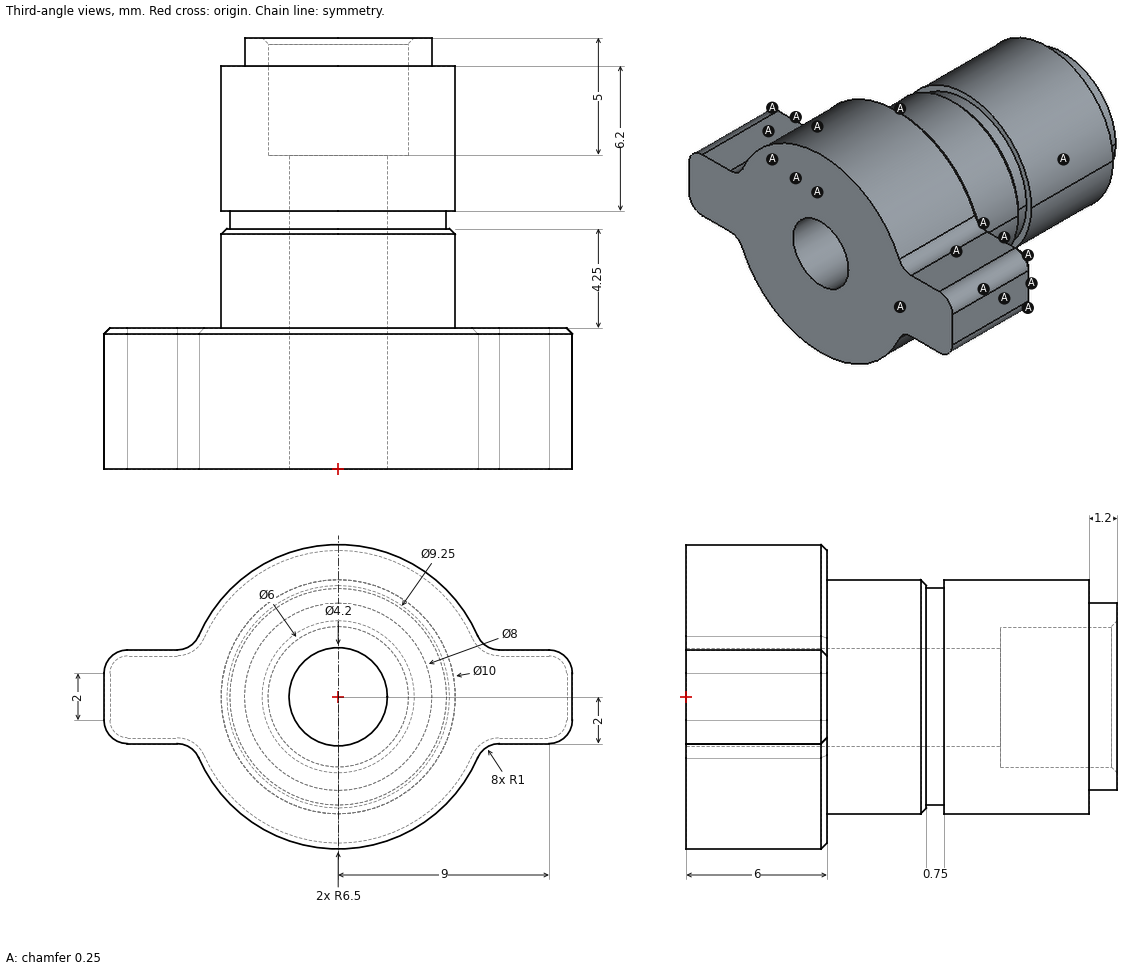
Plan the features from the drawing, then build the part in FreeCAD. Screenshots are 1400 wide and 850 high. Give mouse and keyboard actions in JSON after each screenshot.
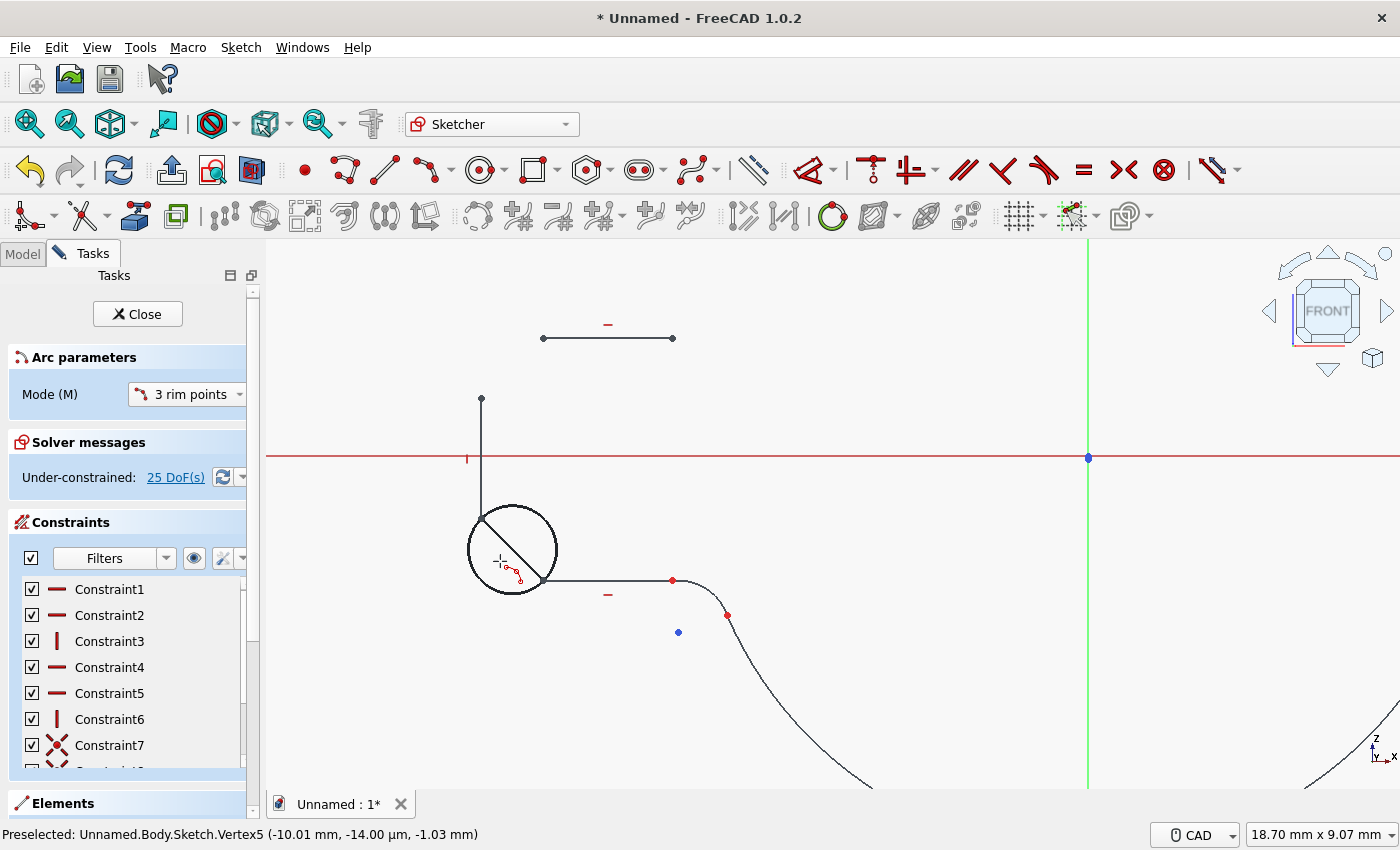
{"action": "left_click", "coordinate": [500, 560]}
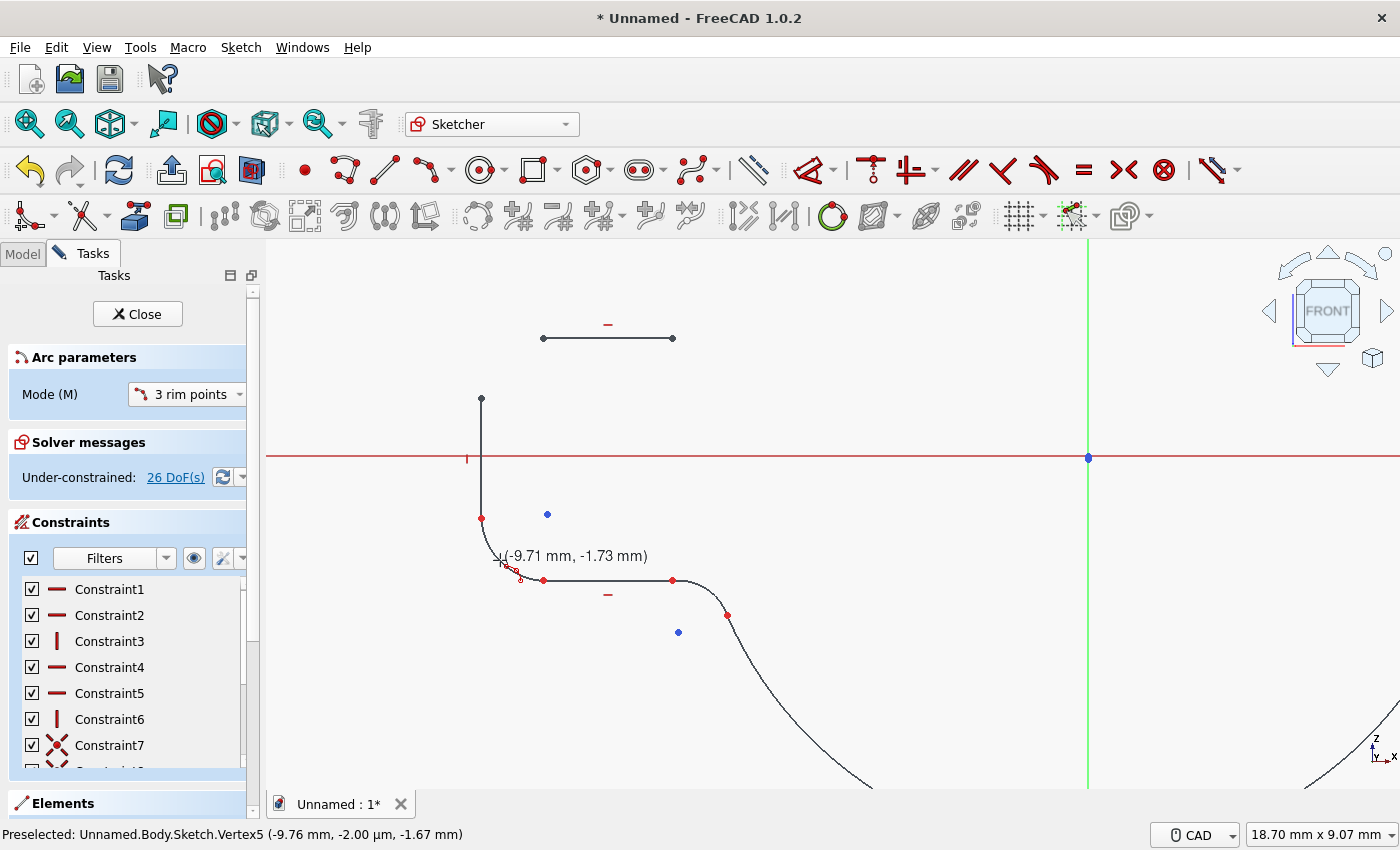
{"action": "left_click", "coordinate": [481, 398]}
{"action": "left_click", "coordinate": [544, 338]}
{"action": "left_click", "coordinate": [500, 353]}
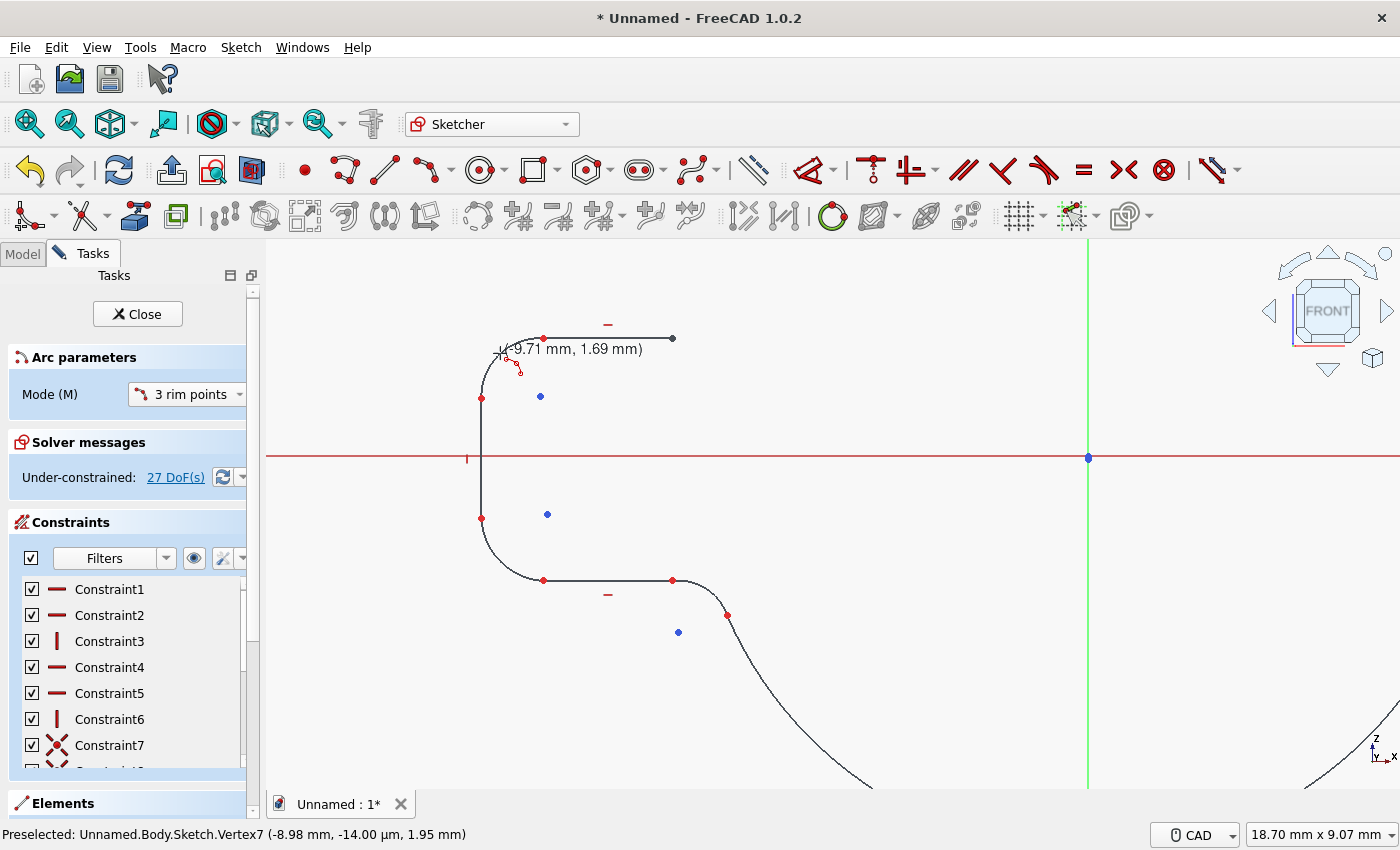
{"action": "left_click", "coordinate": [673, 338]}
{"action": "left_click", "coordinate": [727, 299]}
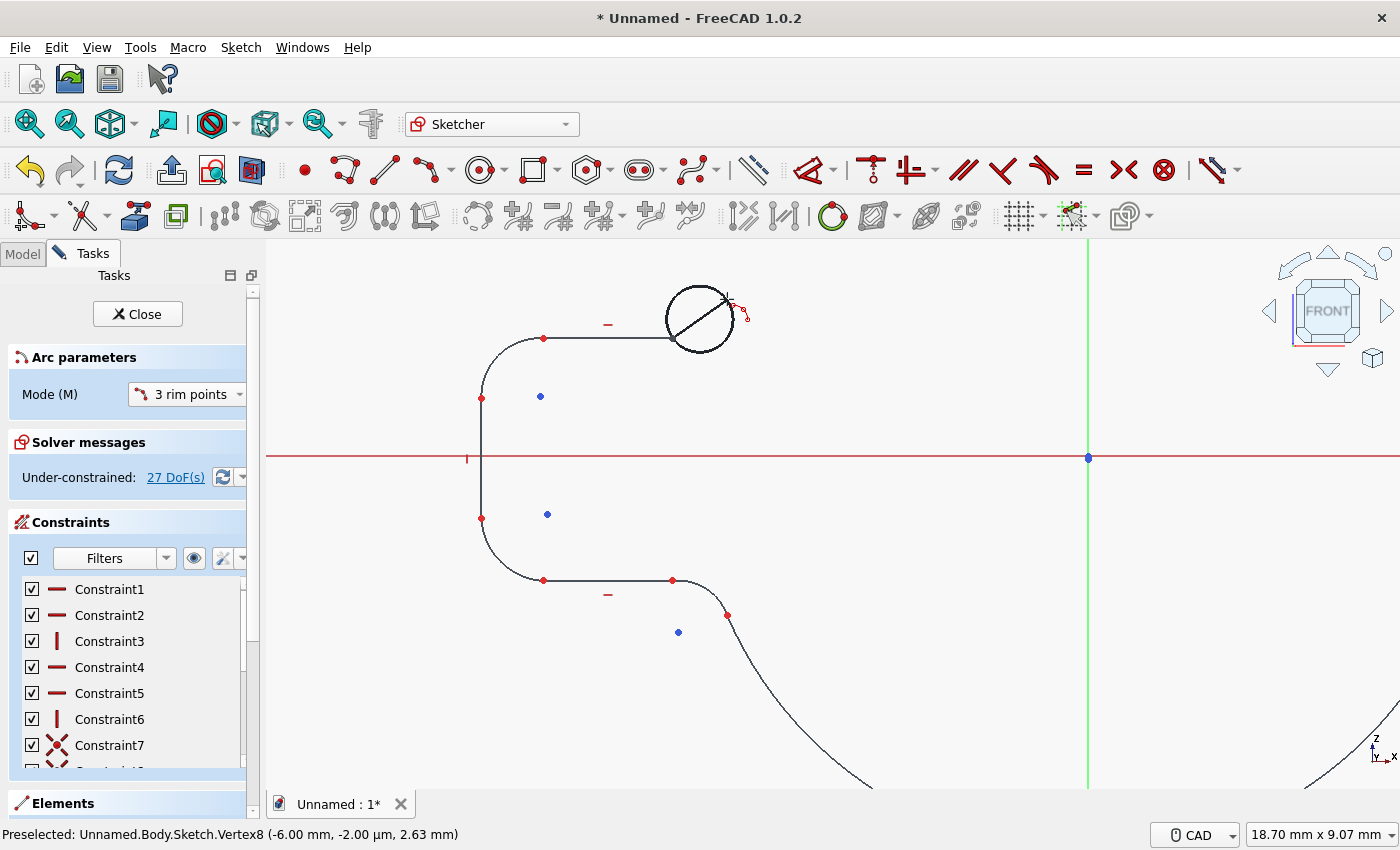
{"action": "scroll", "coordinate": [705, 325], "scroll_direction": "up", "scroll_amount": 3}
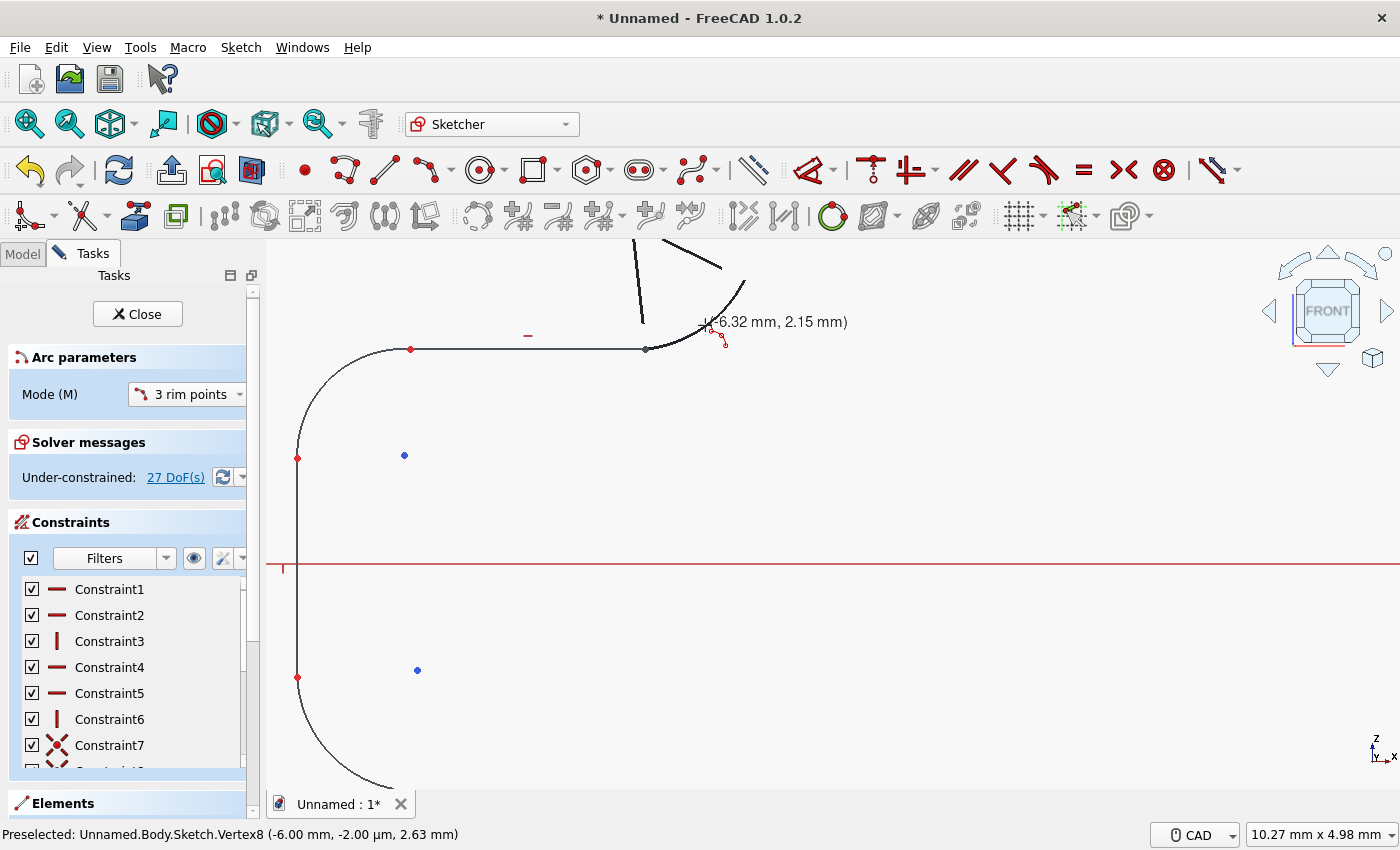
{"action": "left_click", "coordinate": [704, 325]}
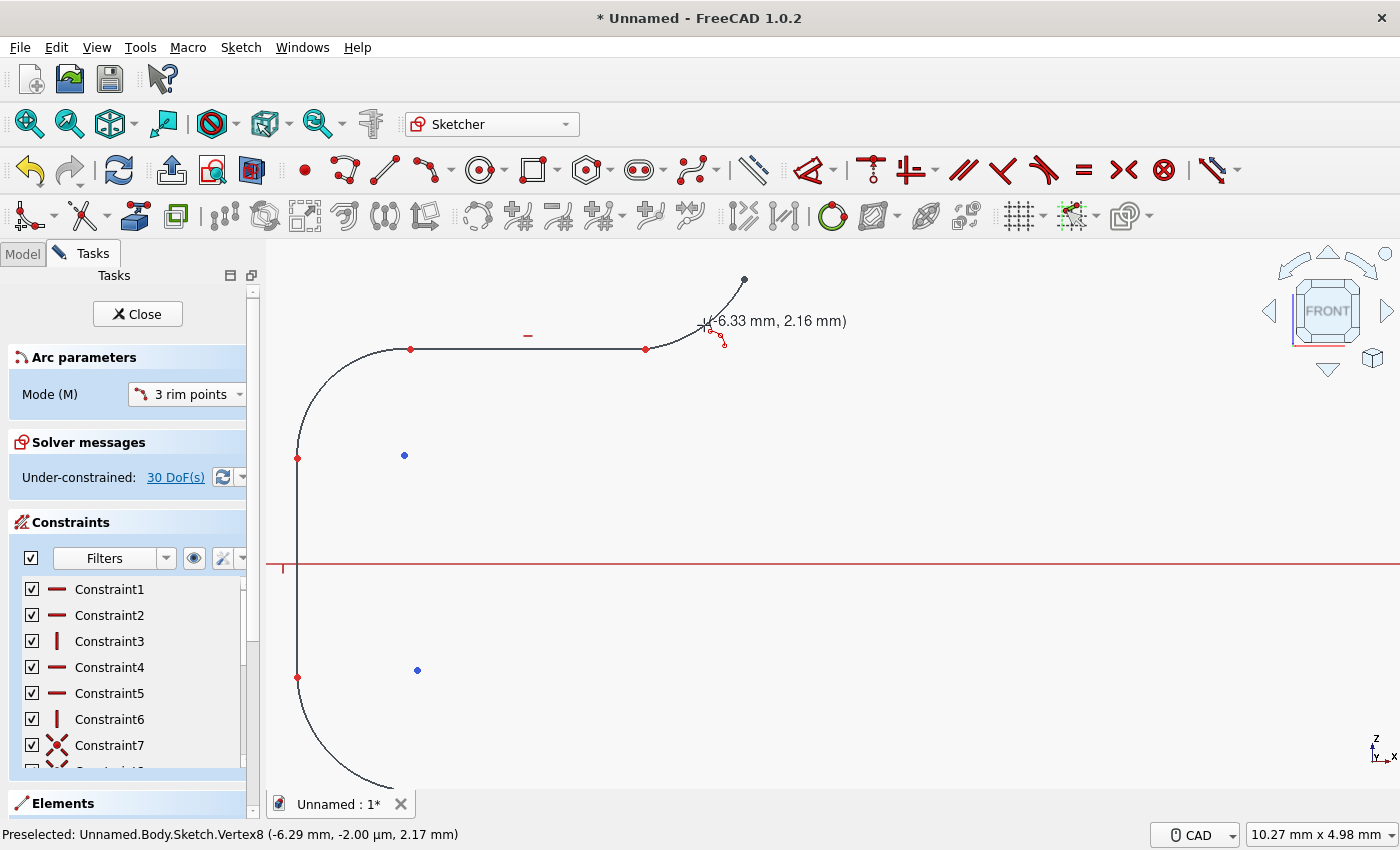
{"action": "scroll", "coordinate": [555, 498], "scroll_direction": "down", "scroll_amount": 7}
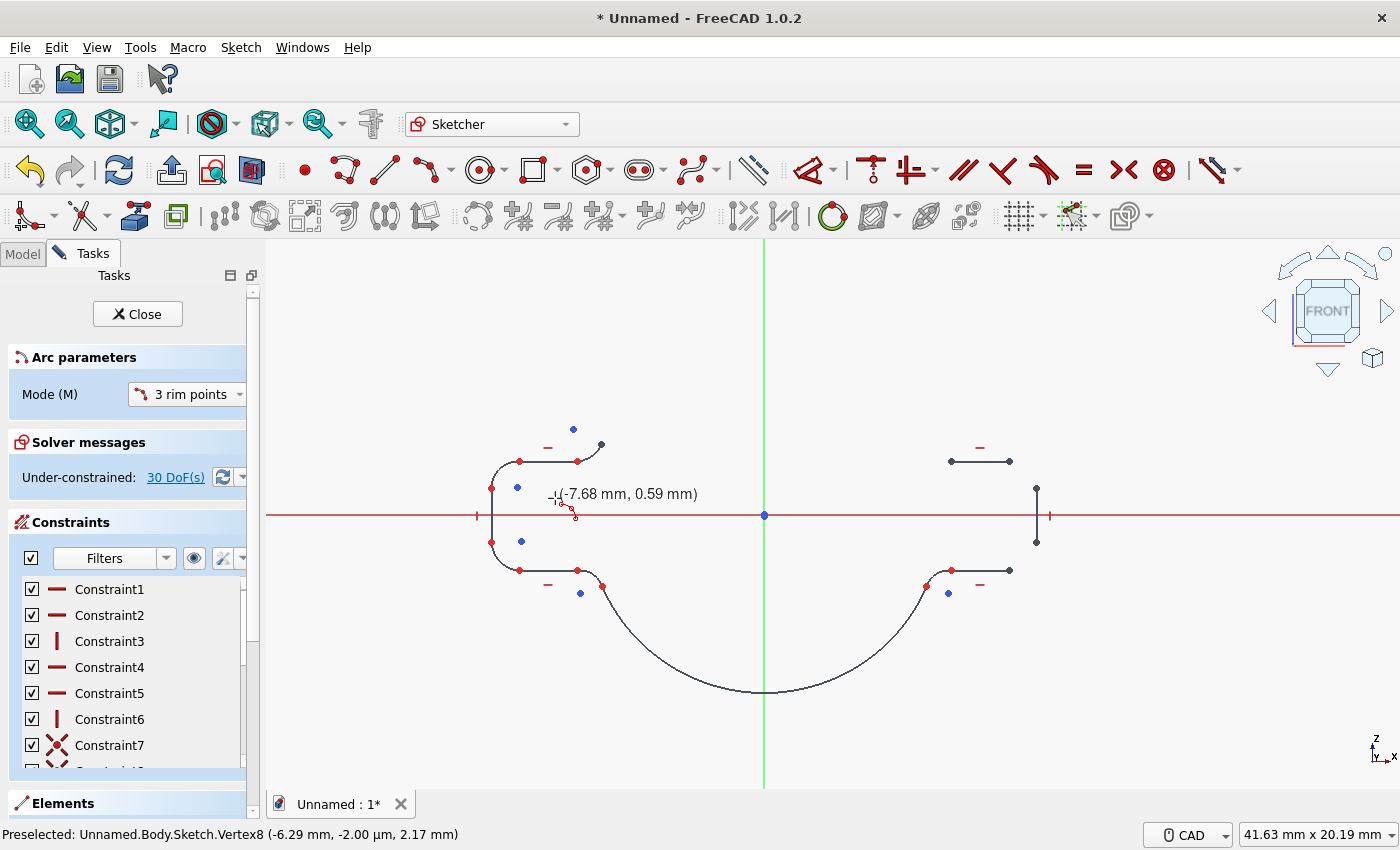
{"action": "left_click", "coordinate": [602, 444]}
{"action": "left_click", "coordinate": [927, 444]}
{"action": "left_click", "coordinate": [805, 342]}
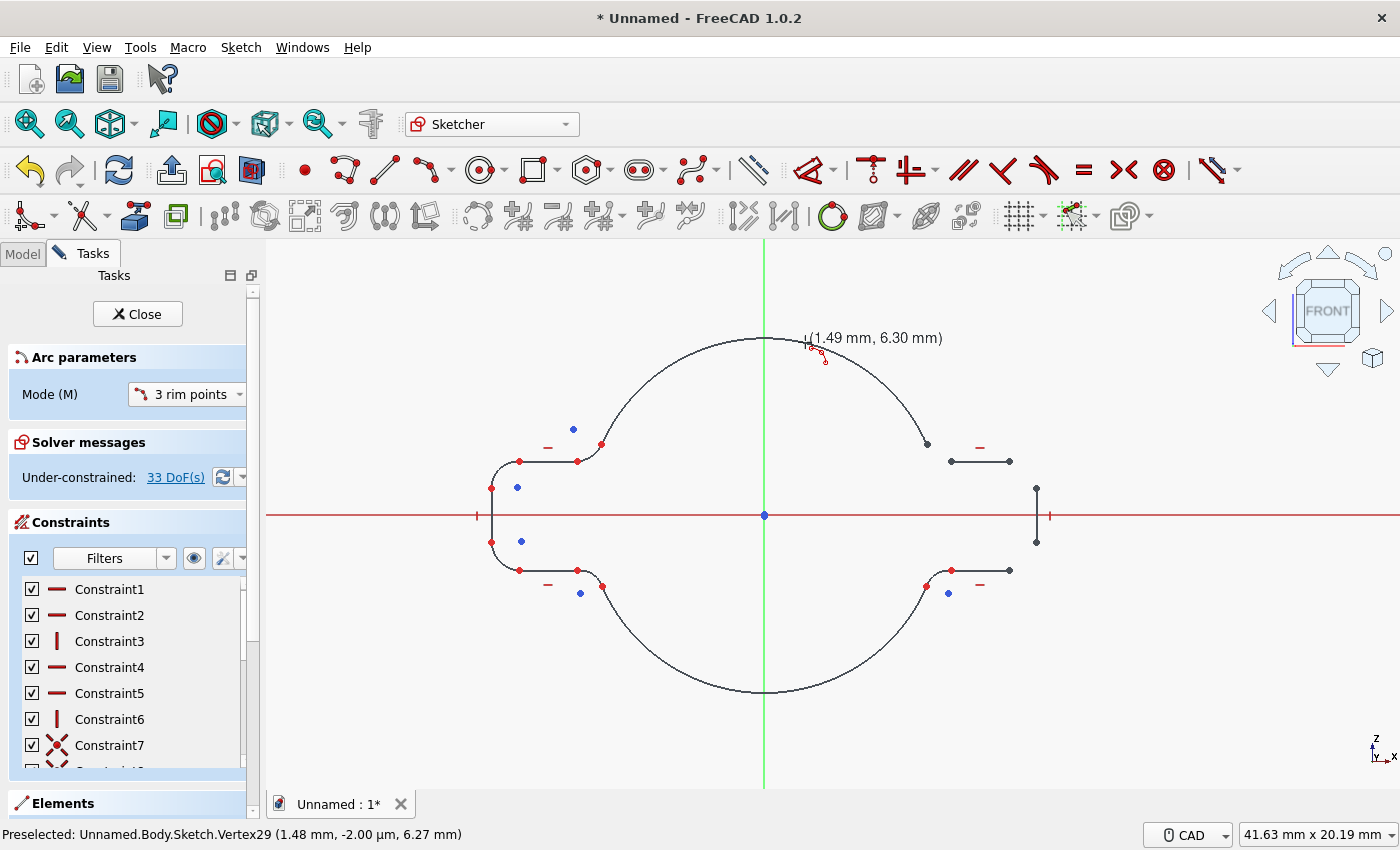
{"action": "left_click", "coordinate": [927, 445]}
{"action": "left_click", "coordinate": [952, 462]}